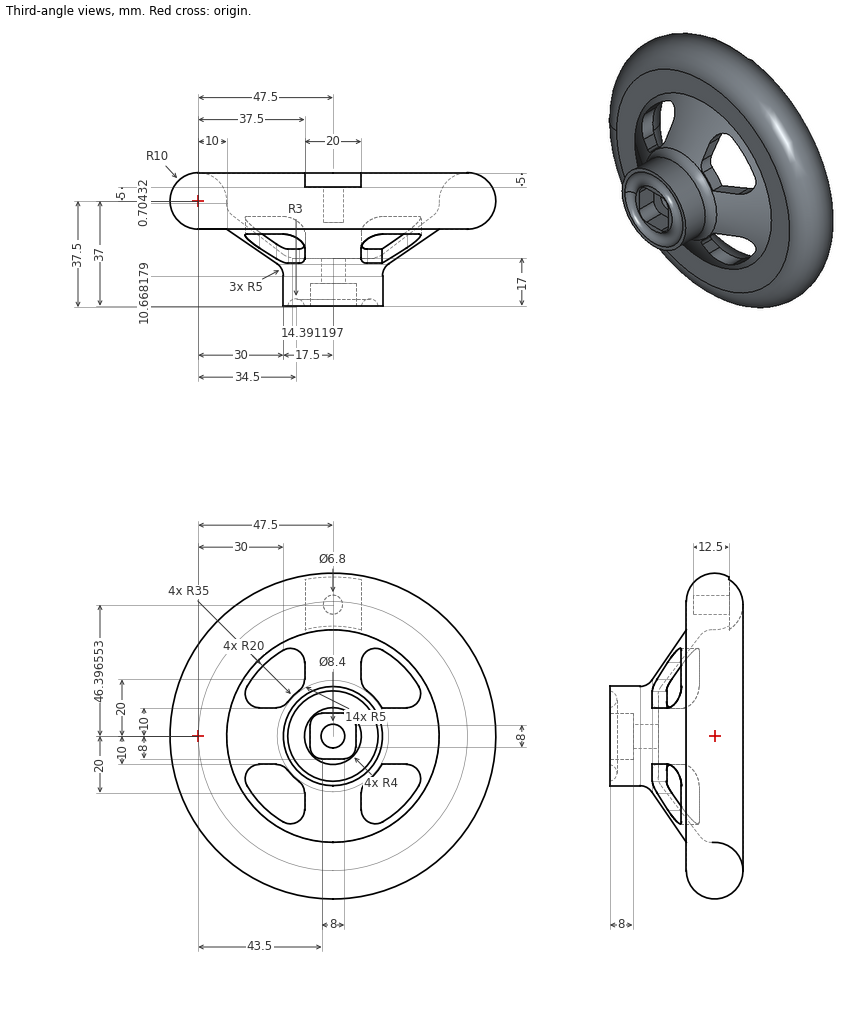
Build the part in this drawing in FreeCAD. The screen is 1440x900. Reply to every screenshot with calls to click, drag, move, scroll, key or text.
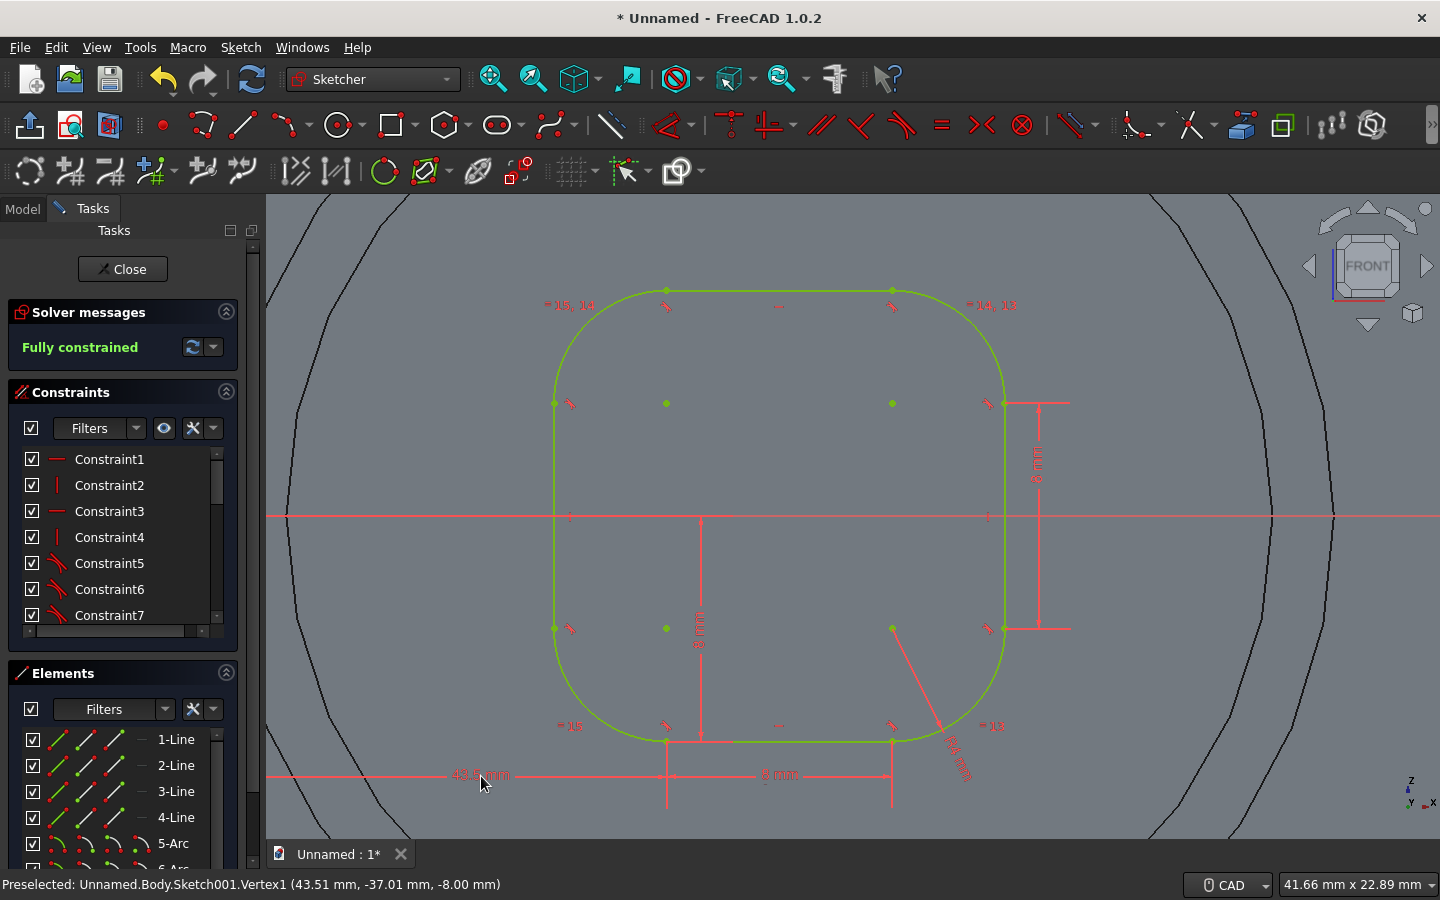
click(123, 269)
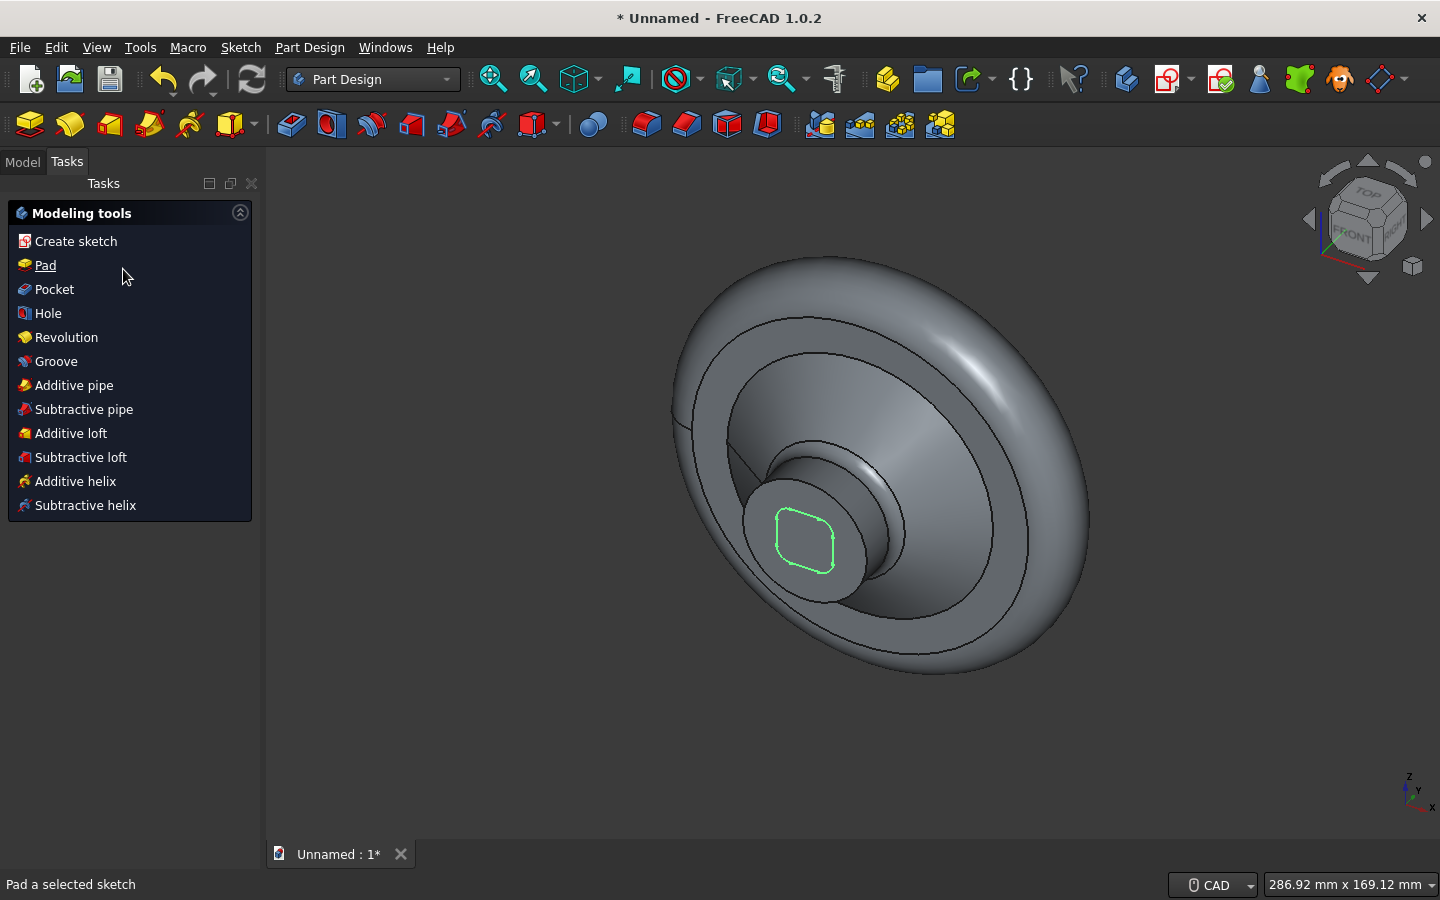
click(292, 124)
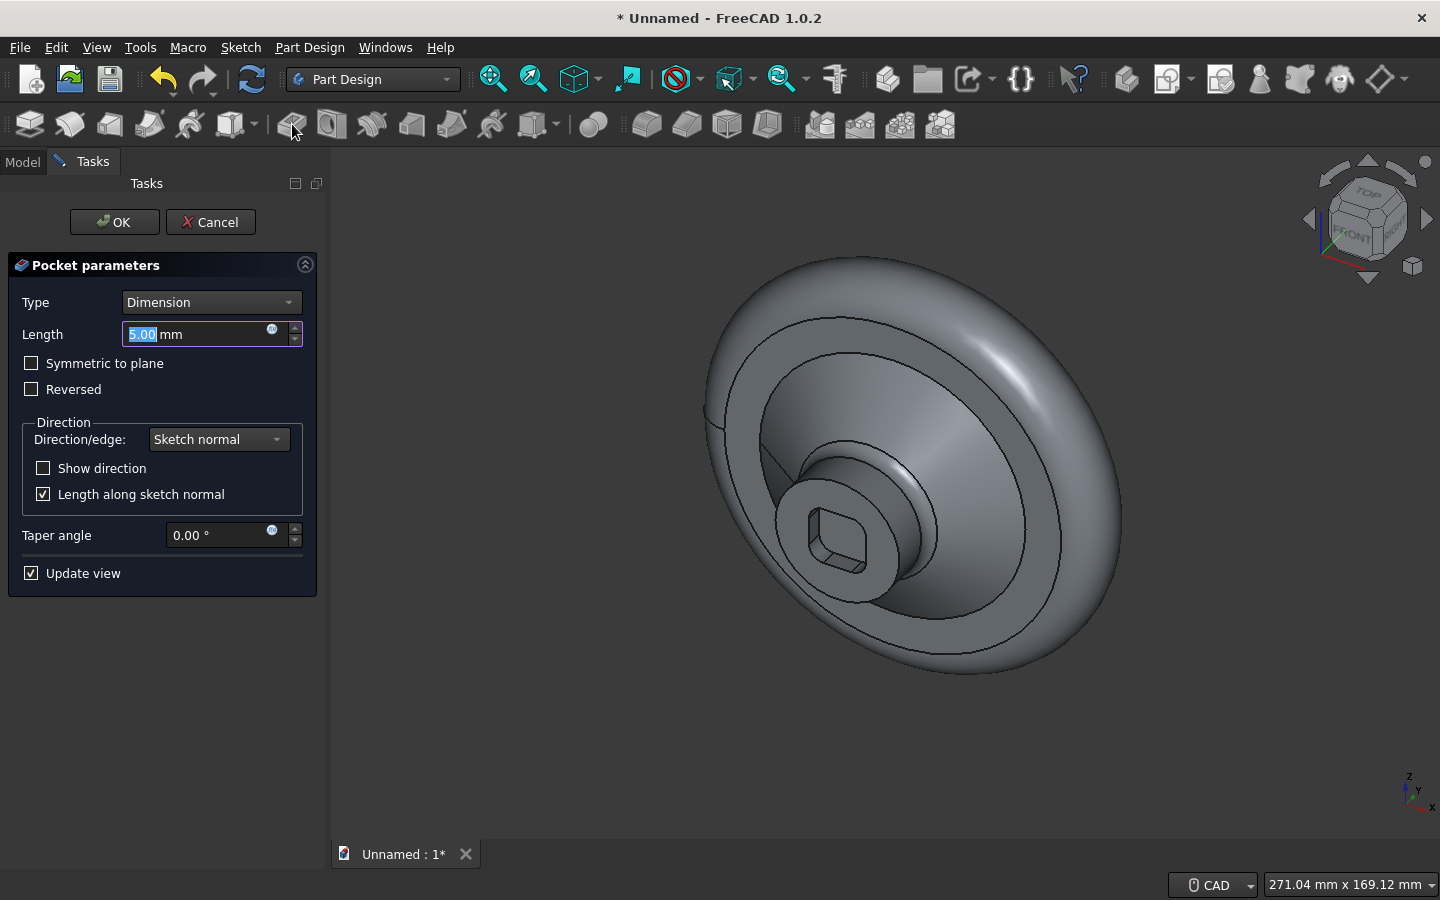
text(8)
key(Tab)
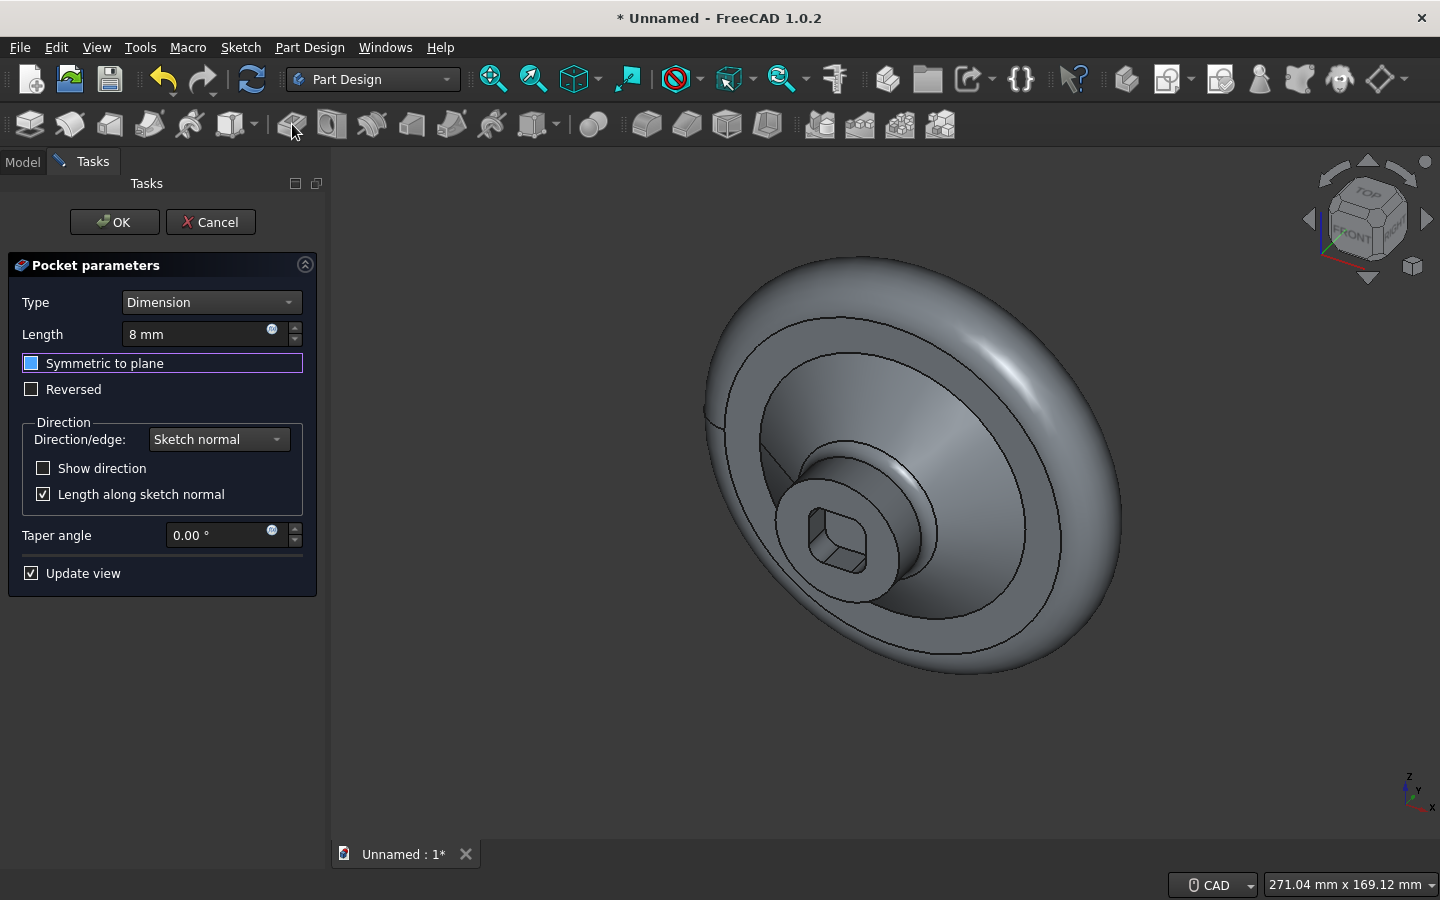
click(115, 222)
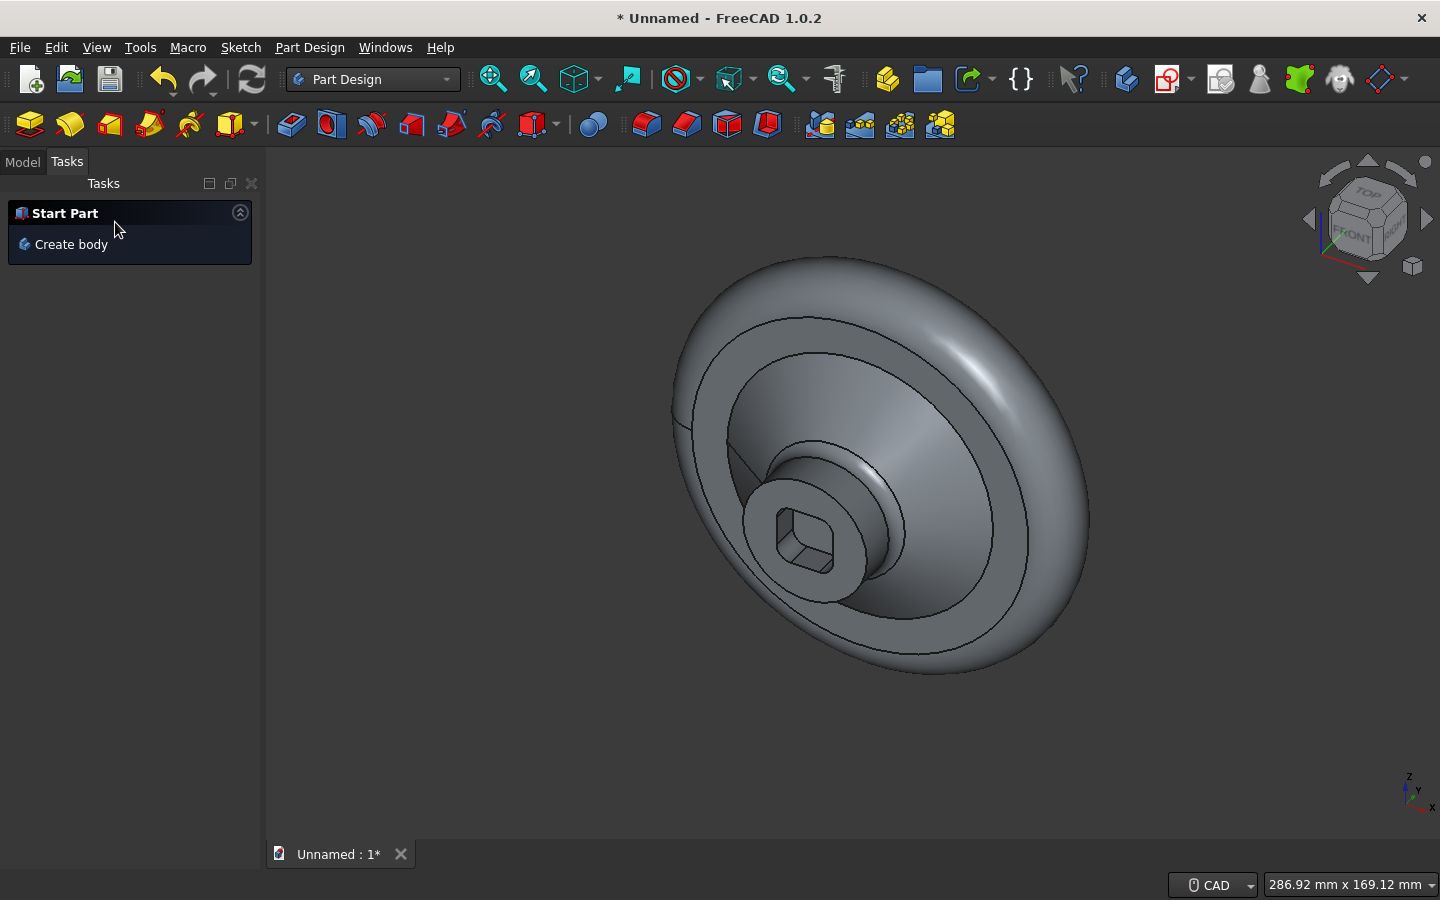
click(769, 561)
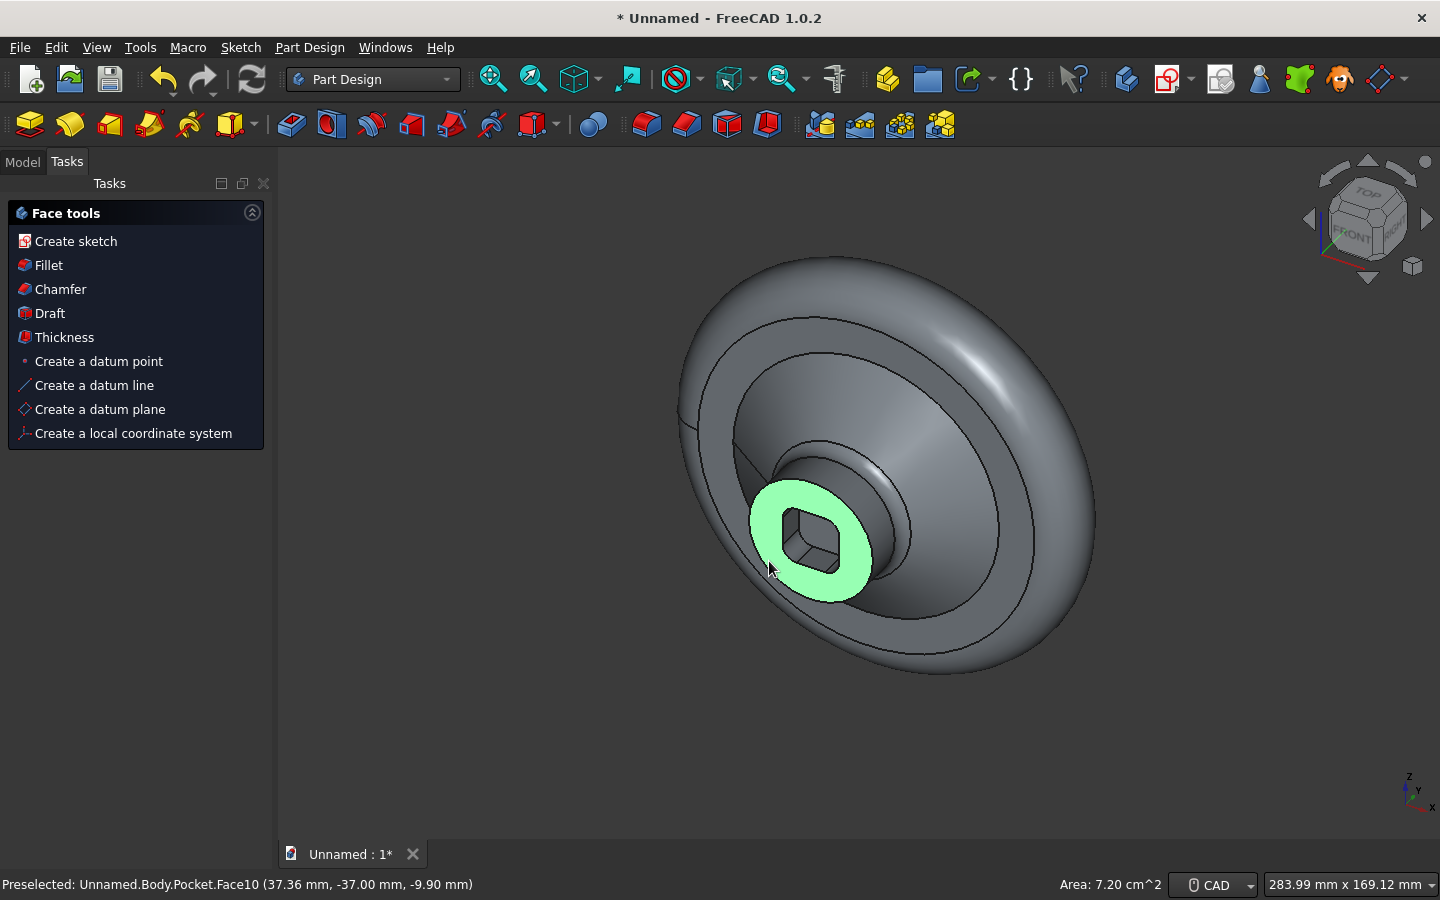
click(1168, 80)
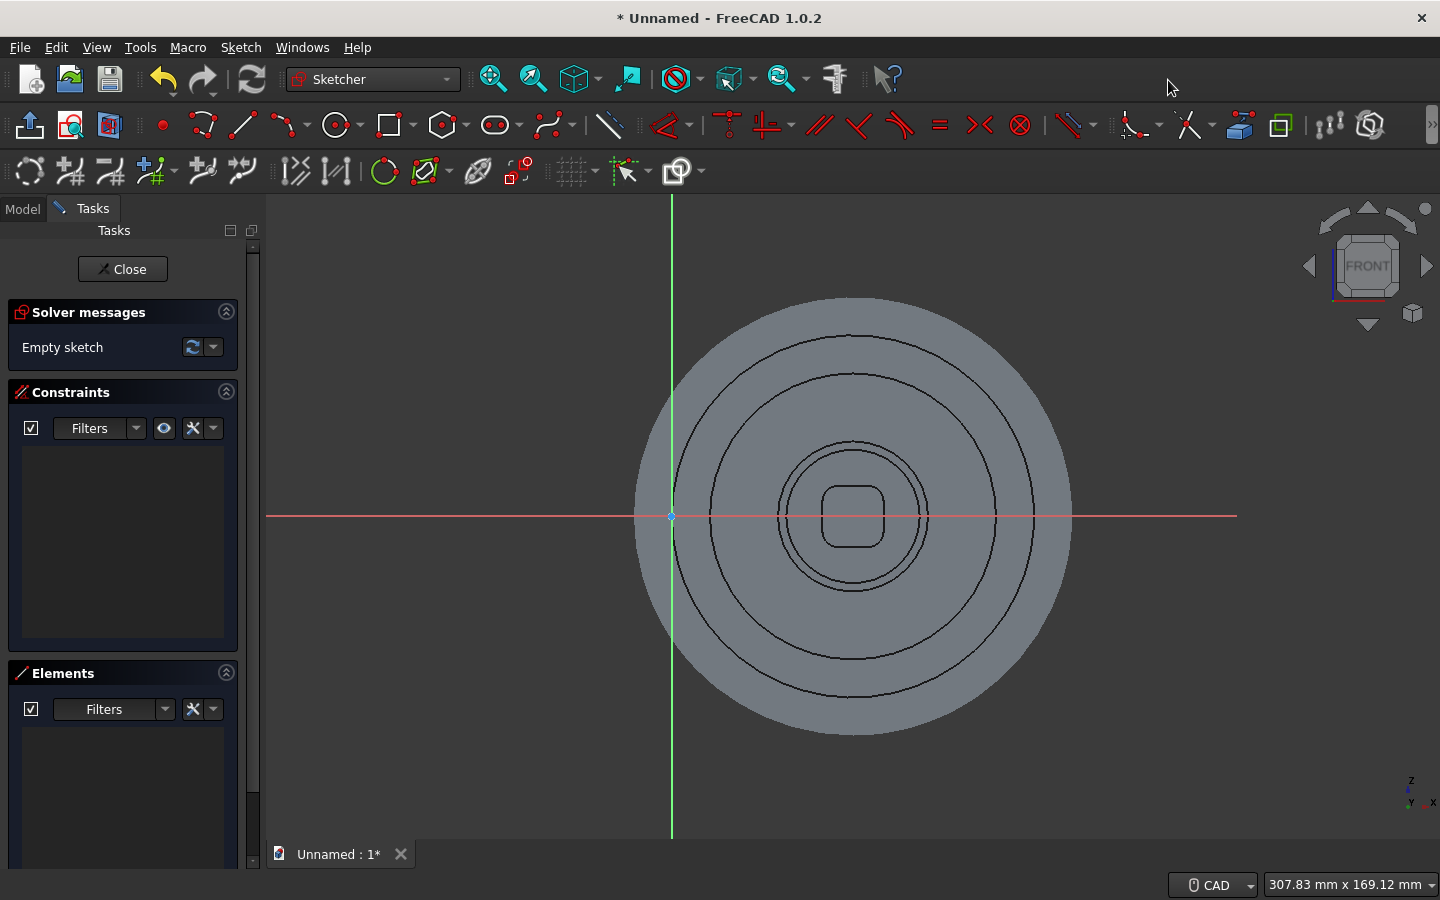
scroll(858, 516, up, 13)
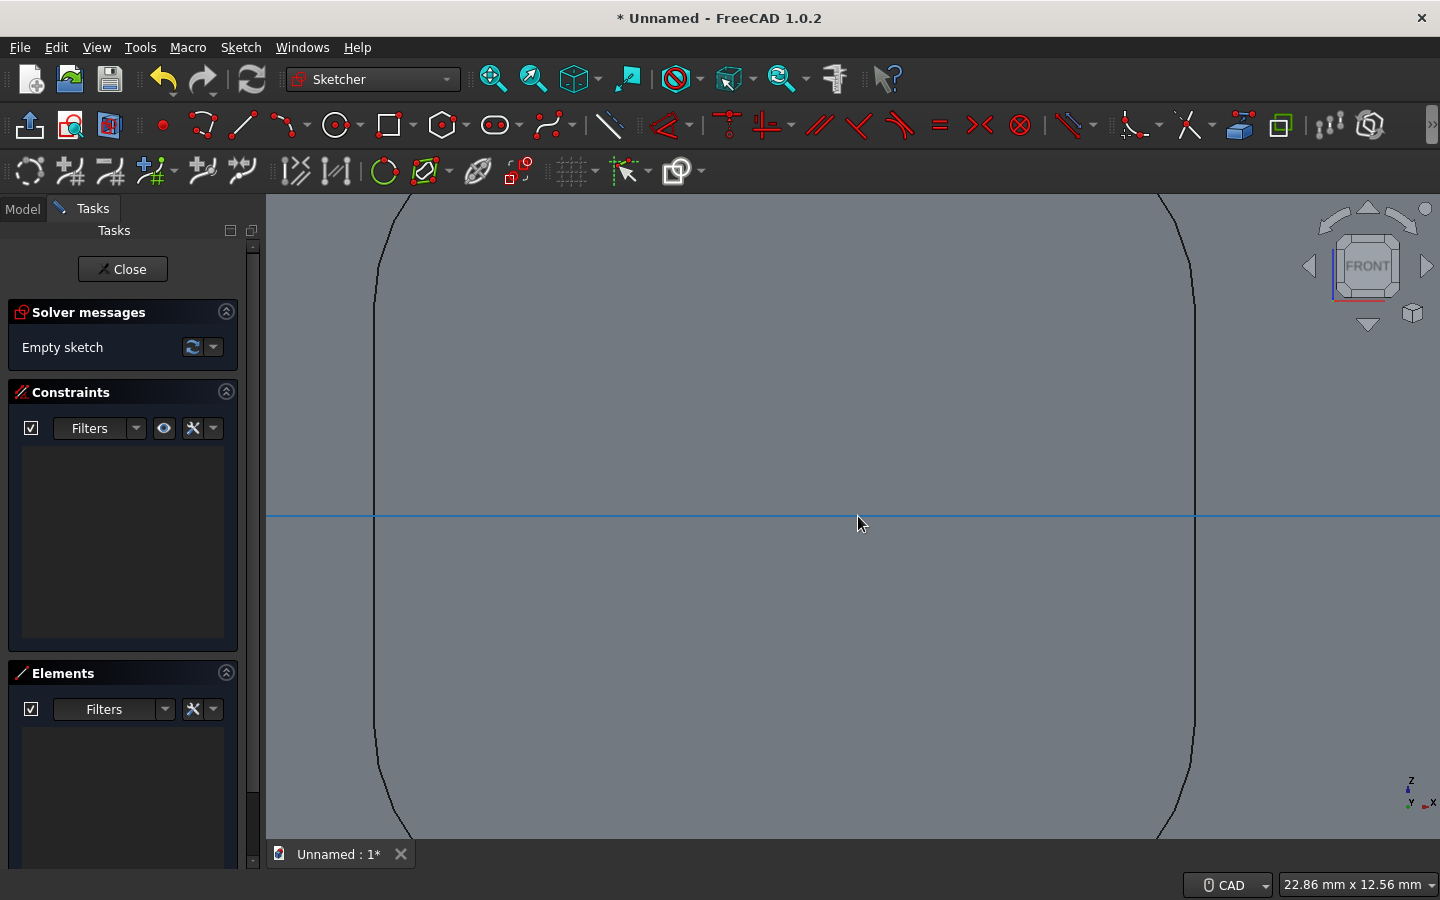
click(336, 126)